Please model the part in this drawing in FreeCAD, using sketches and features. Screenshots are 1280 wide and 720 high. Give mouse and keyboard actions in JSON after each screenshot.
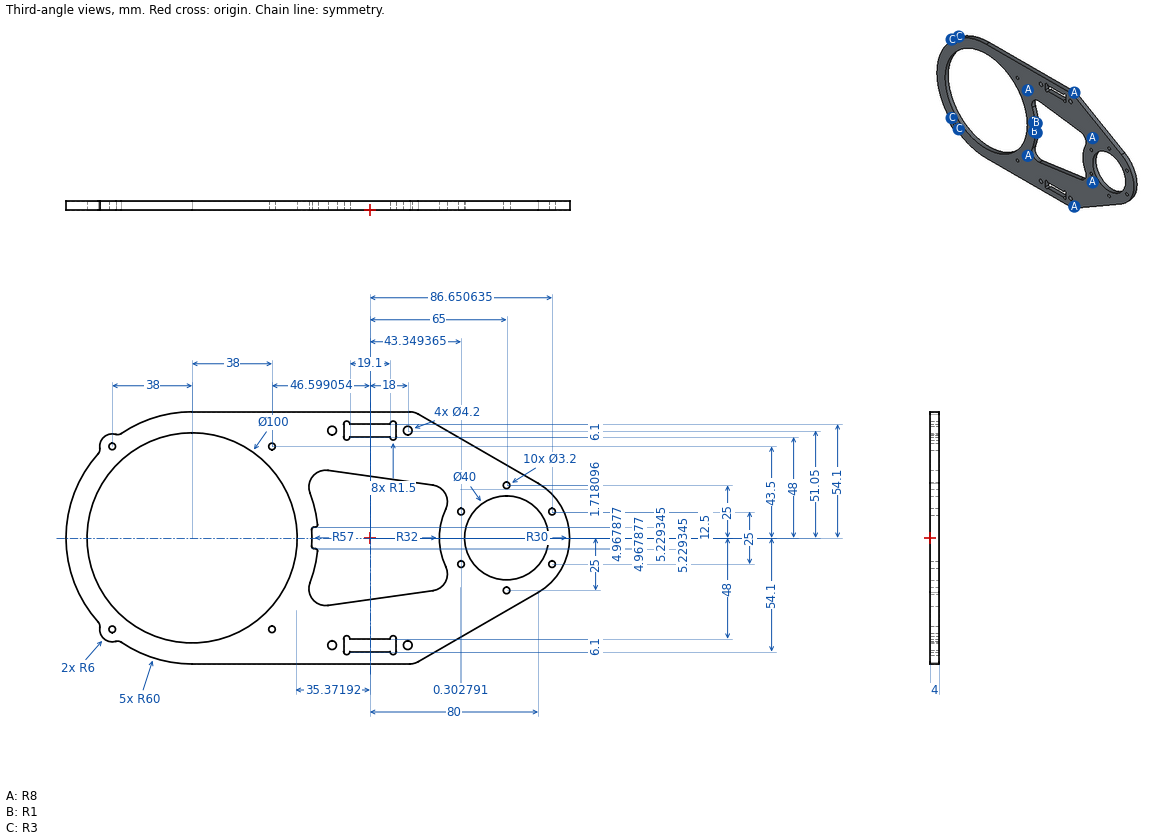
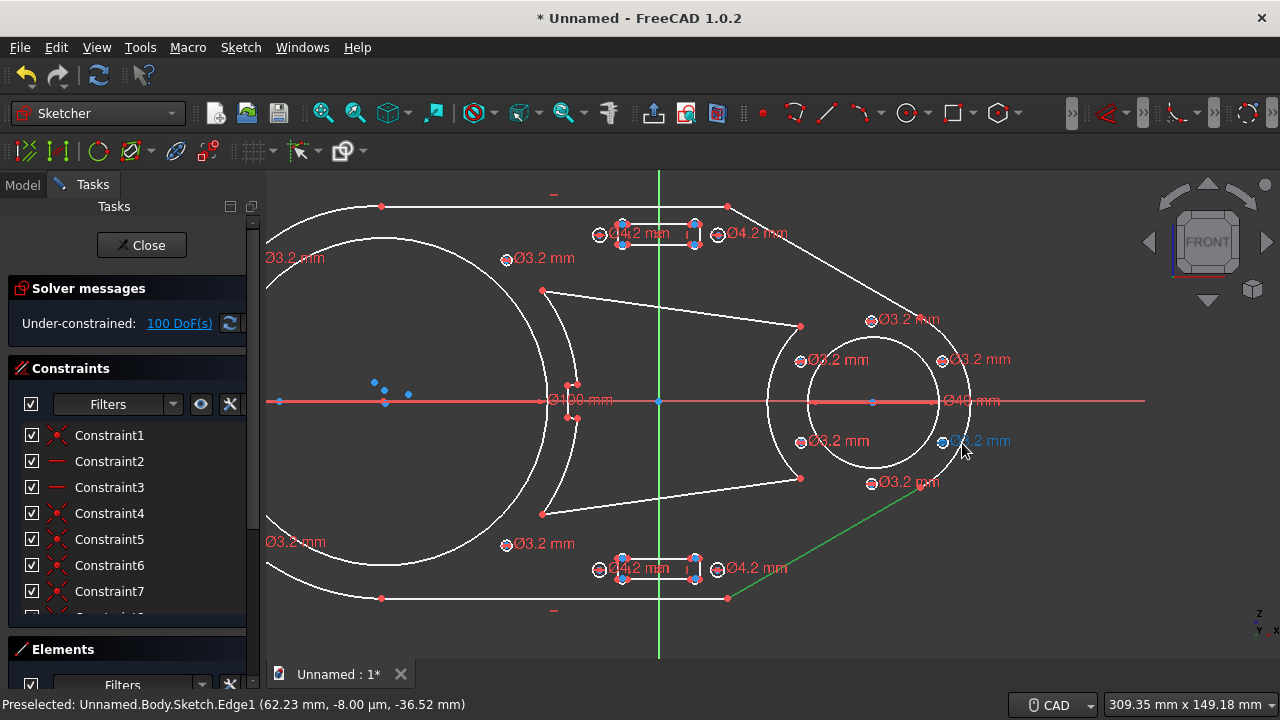
{"action": "left_click", "coordinate": [952, 460]}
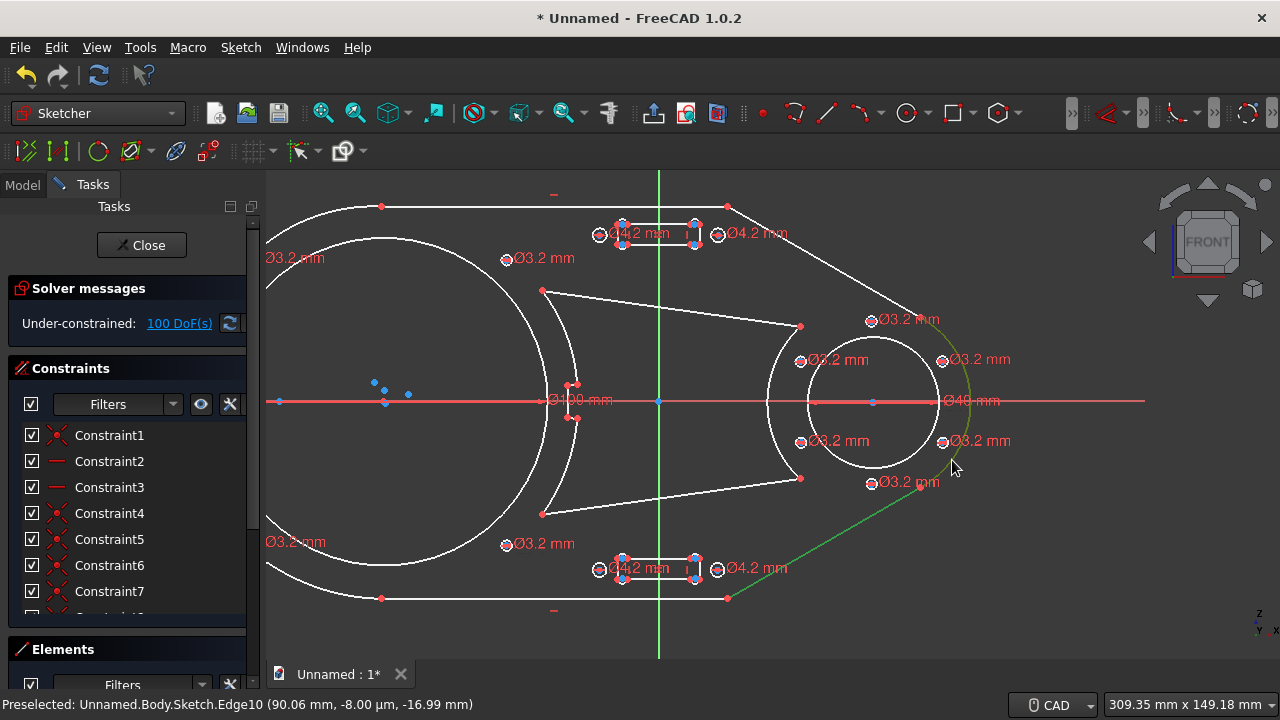
{"action": "key", "text": "t"}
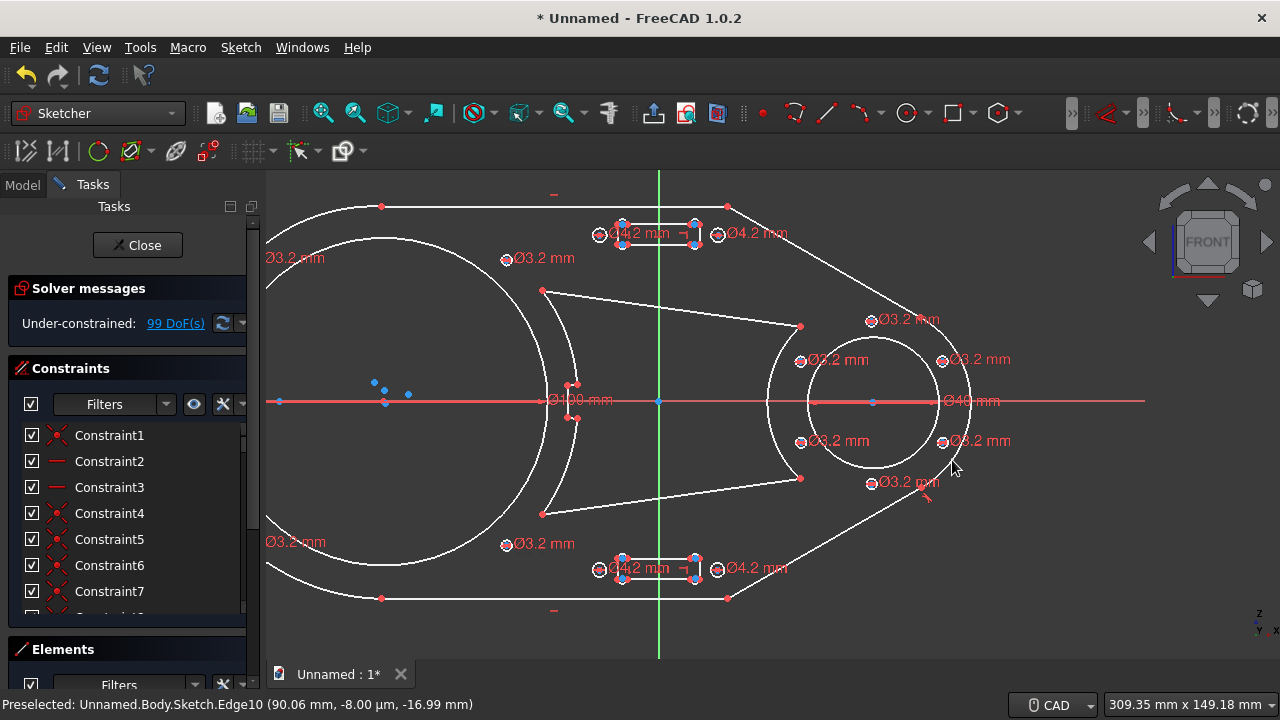
{"action": "left_click", "coordinate": [786, 240]}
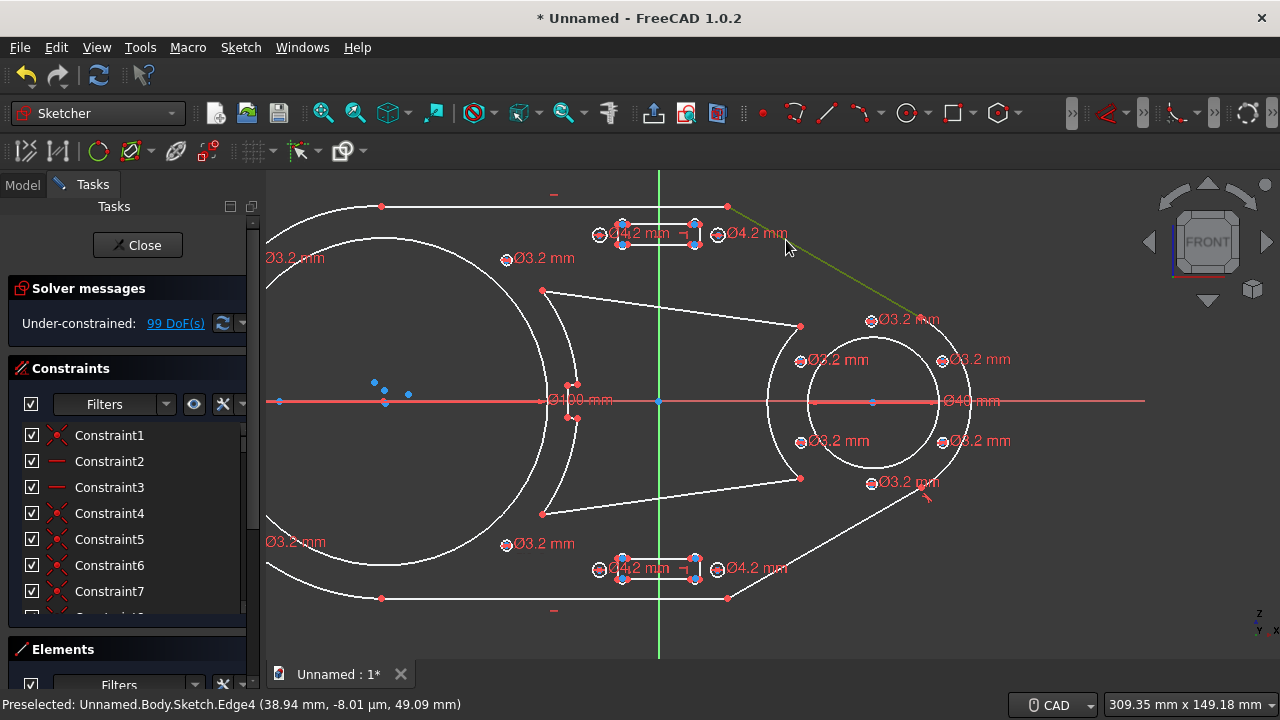
{"action": "left_click", "coordinate": [952, 460]}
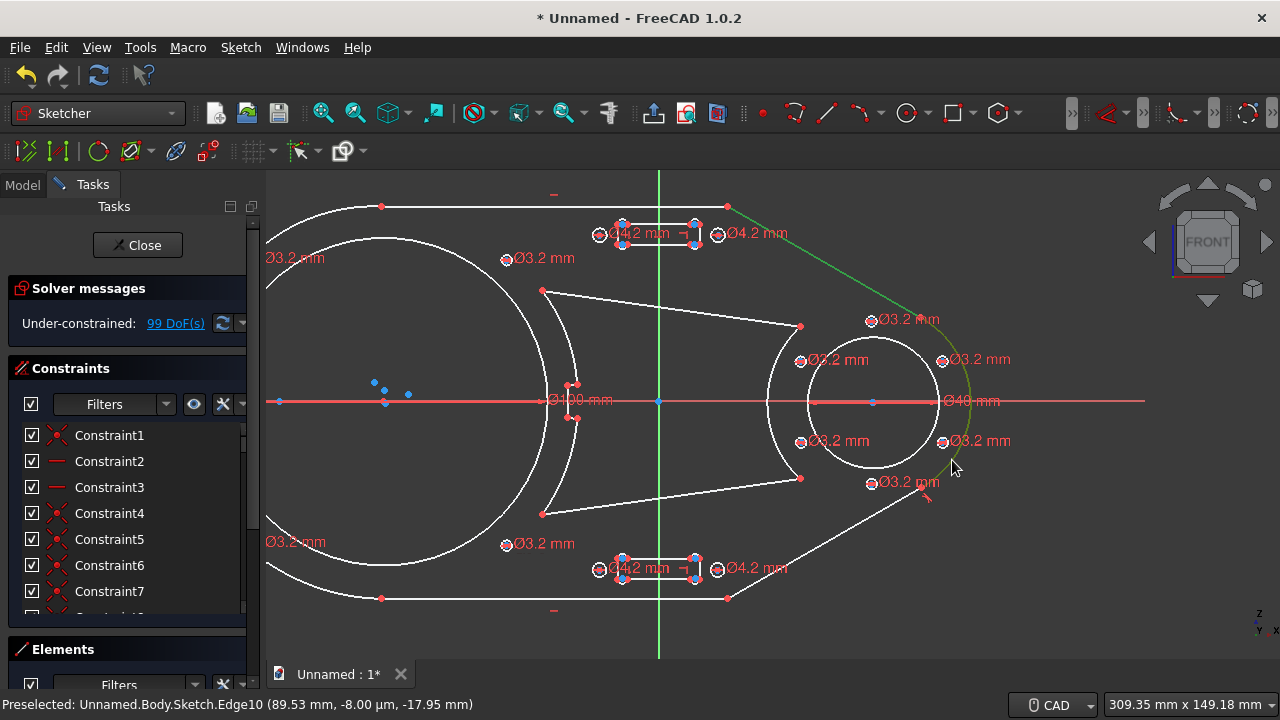
{"action": "key", "text": "t"}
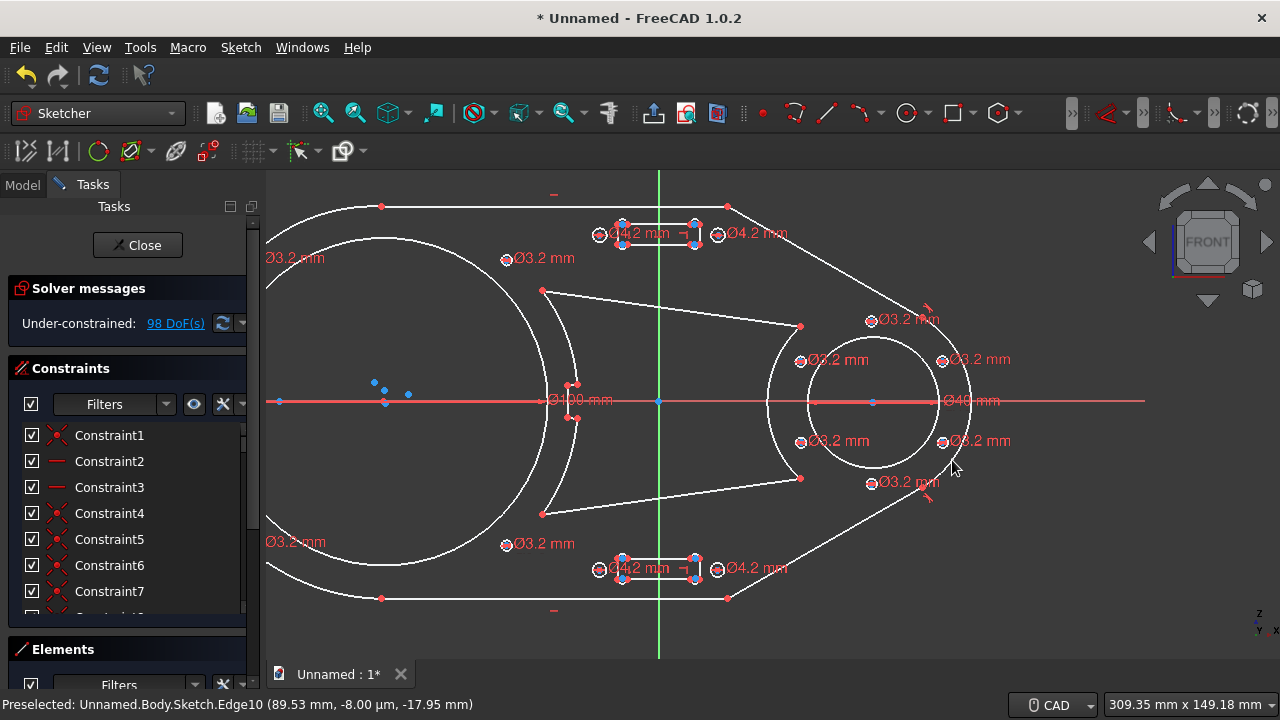
{"action": "scroll", "coordinate": [700, 234], "scroll_direction": "up", "scroll_amount": 2}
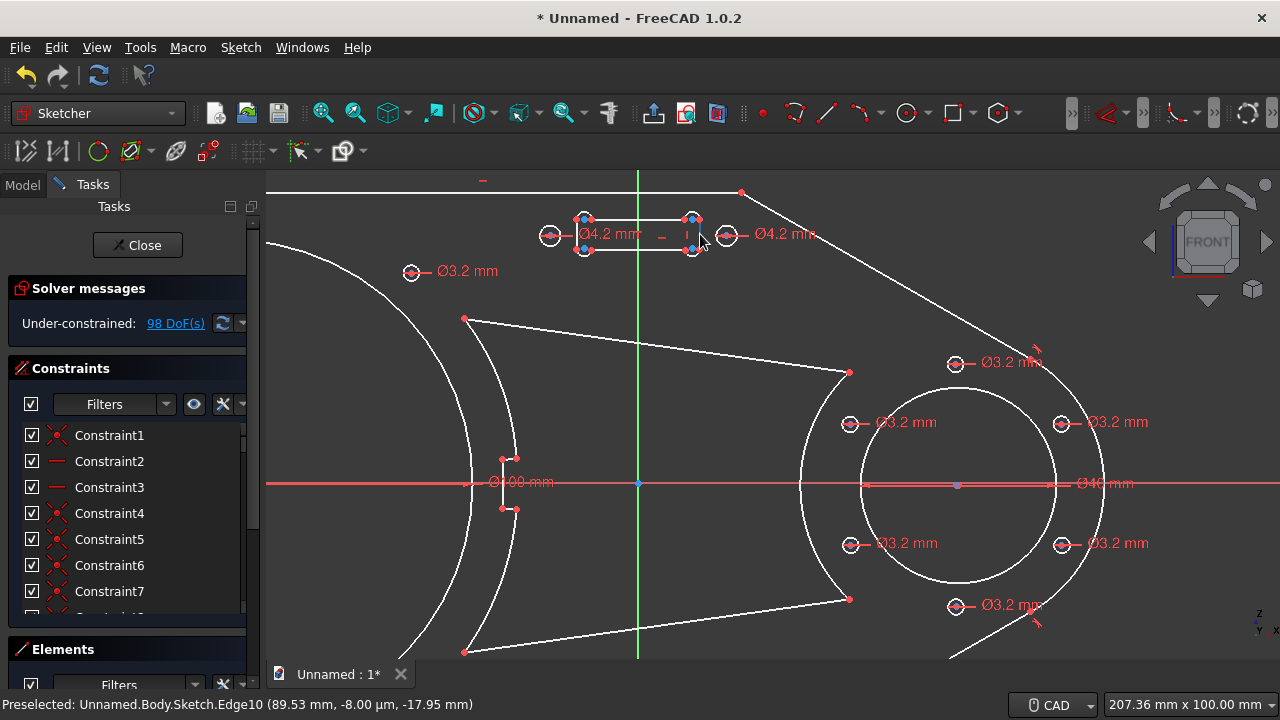
{"action": "left_click", "coordinate": [700, 234]}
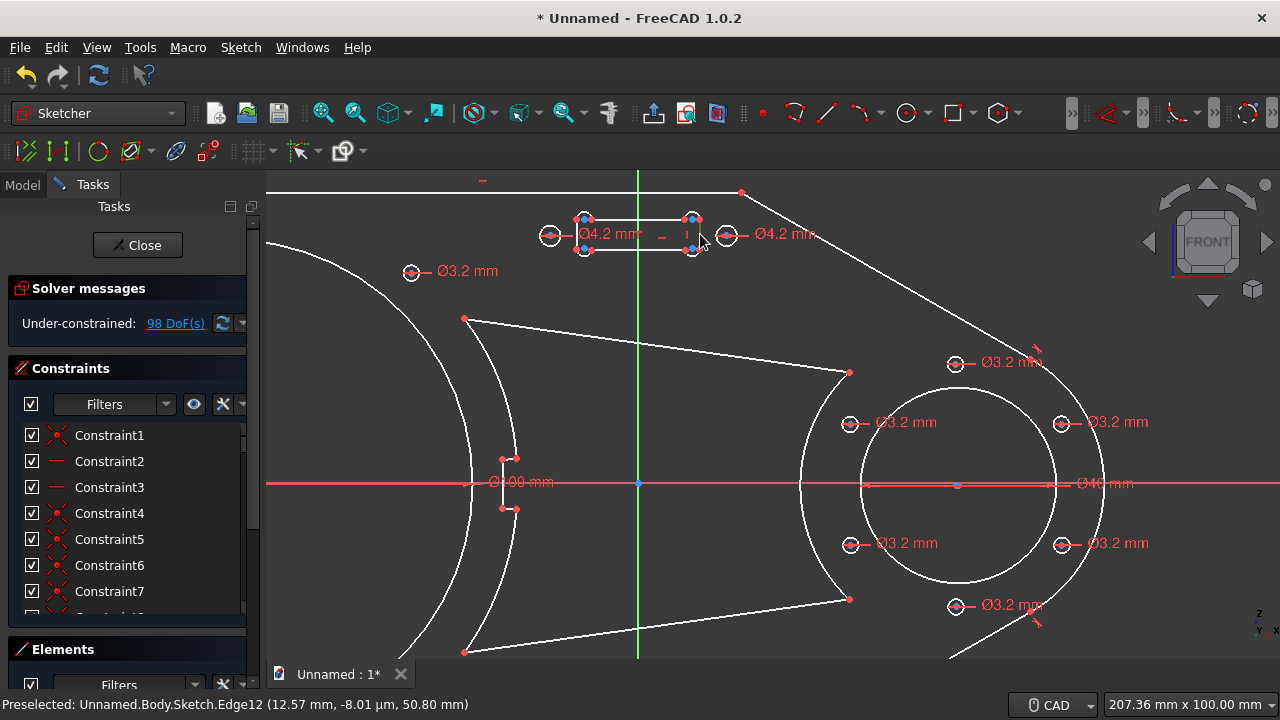
{"action": "scroll", "coordinate": [693, 256], "scroll_direction": "up", "scroll_amount": 4}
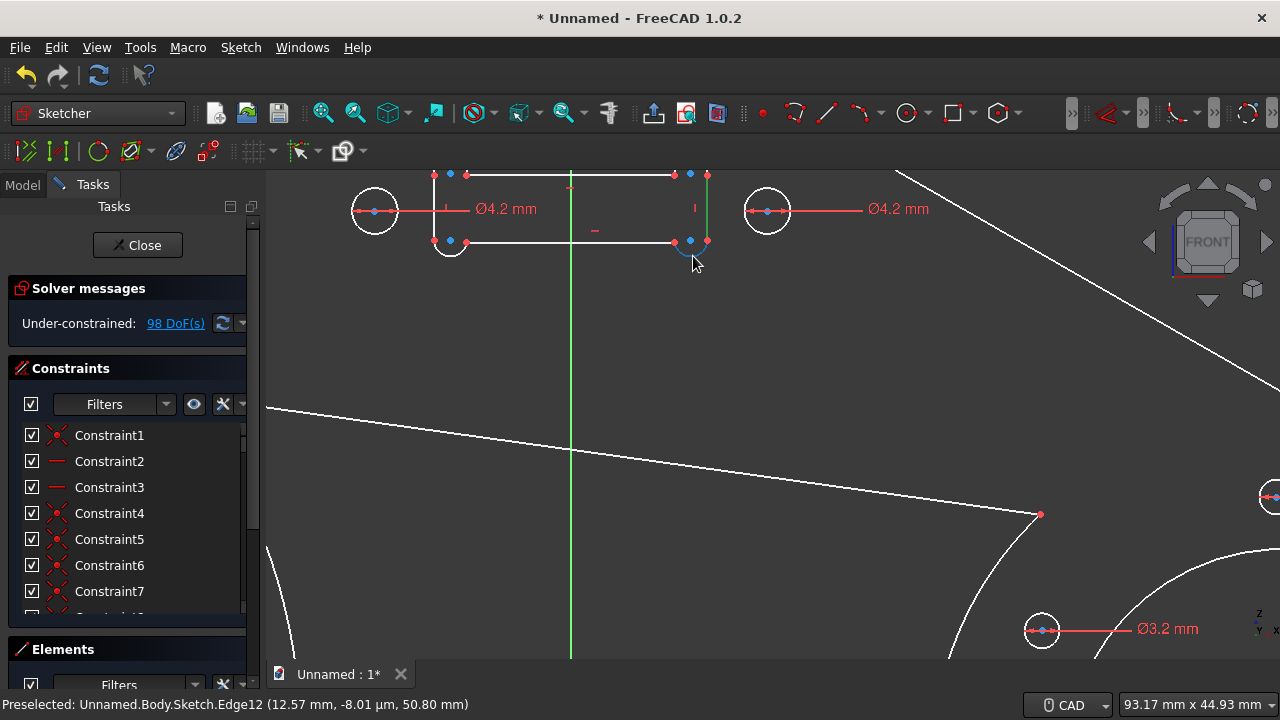
{"action": "left_click", "coordinate": [692, 256]}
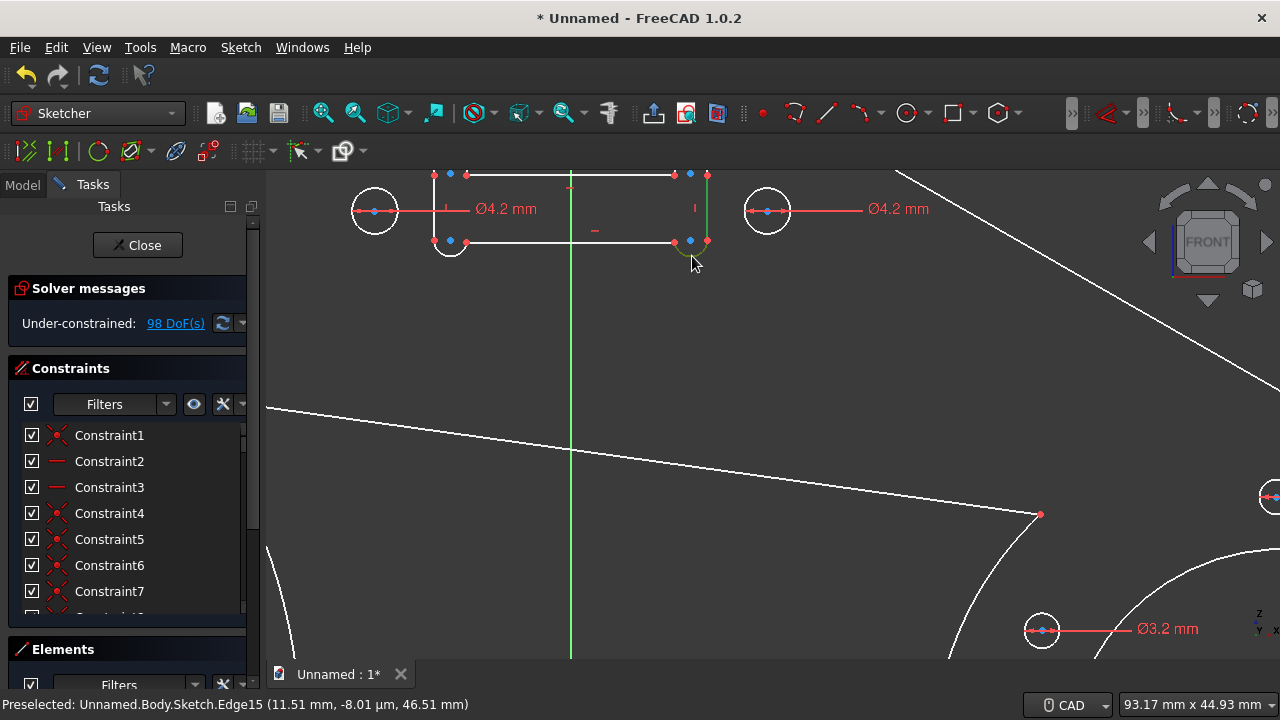
{"action": "key", "text": "t"}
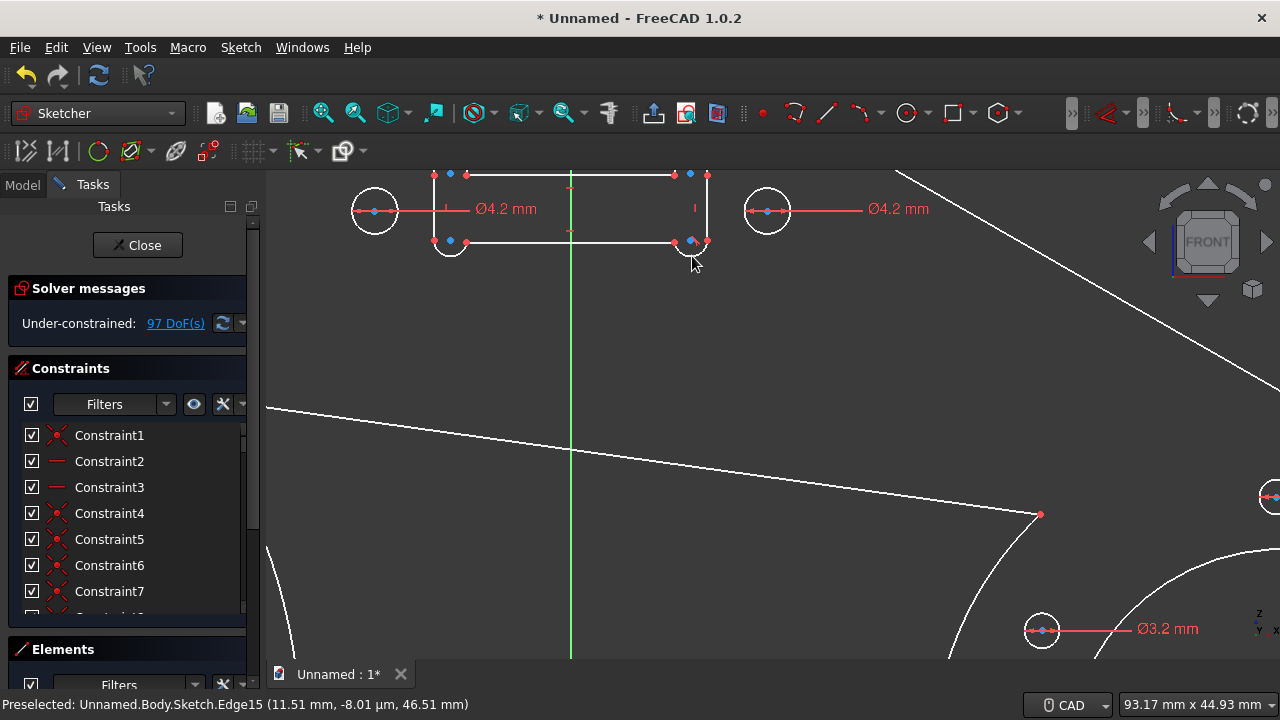
{"action": "left_click", "coordinate": [707, 221]}